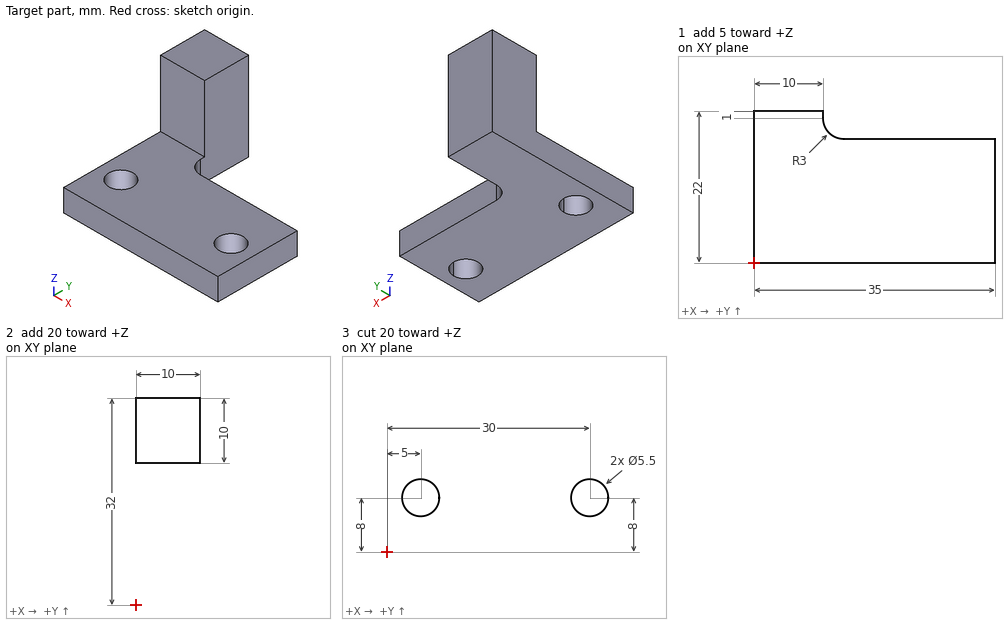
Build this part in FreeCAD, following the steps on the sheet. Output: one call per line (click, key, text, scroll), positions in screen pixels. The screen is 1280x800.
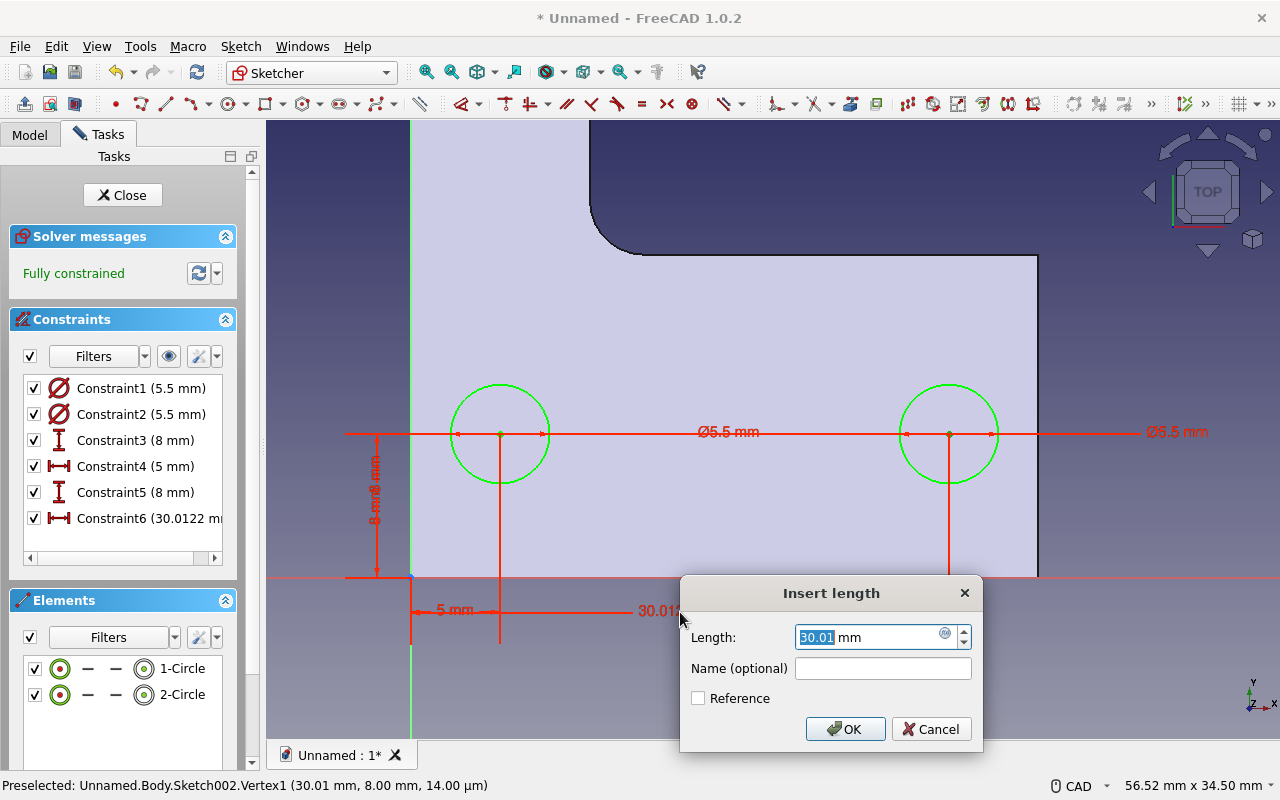
text(30)
key(Return)
key(Escape)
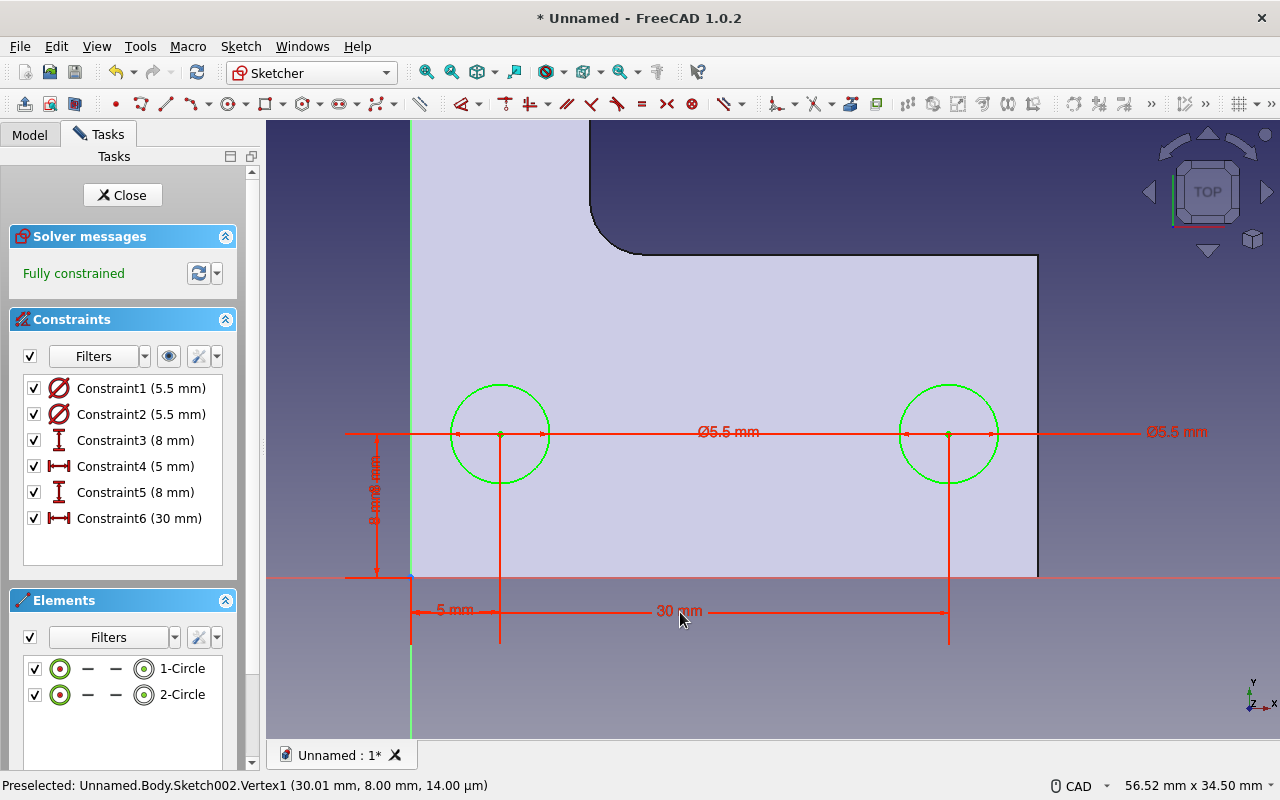
click(123, 195)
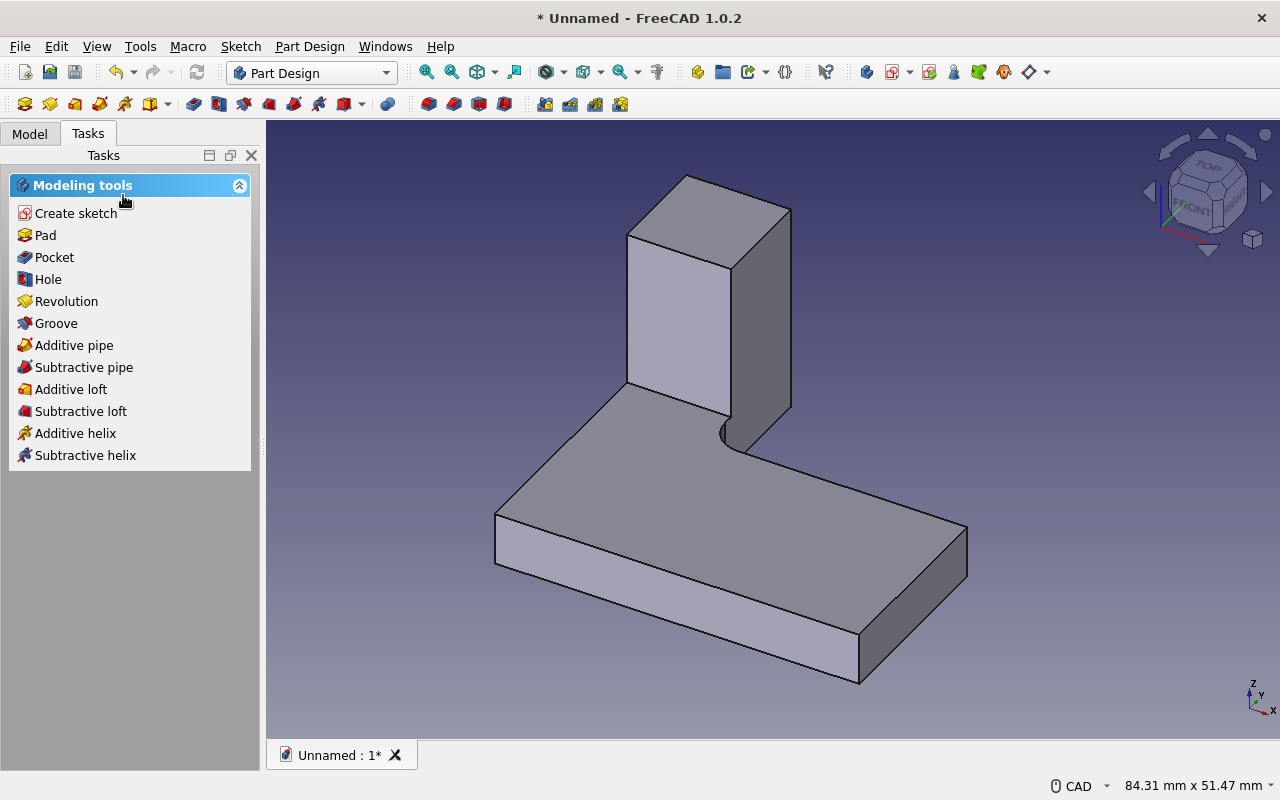
click(194, 104)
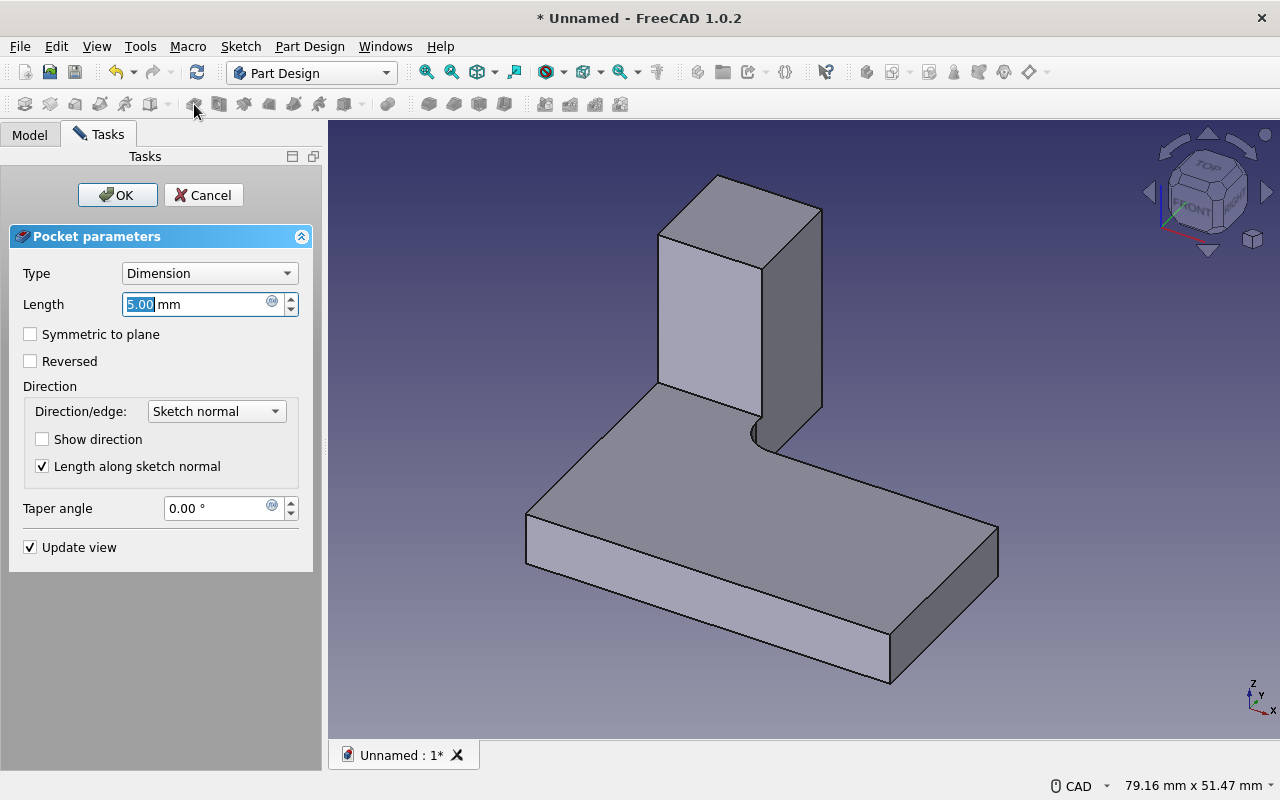
text(20)
key(Tab)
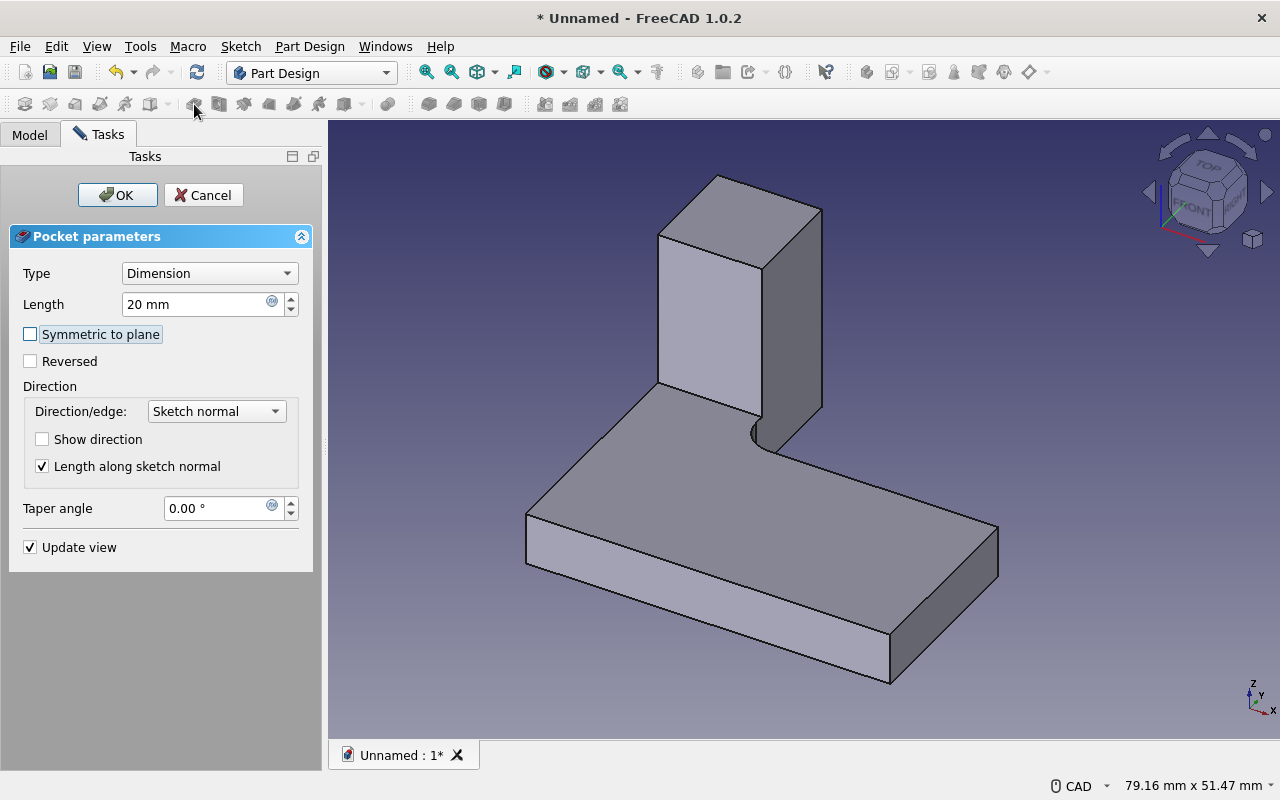
click(31, 361)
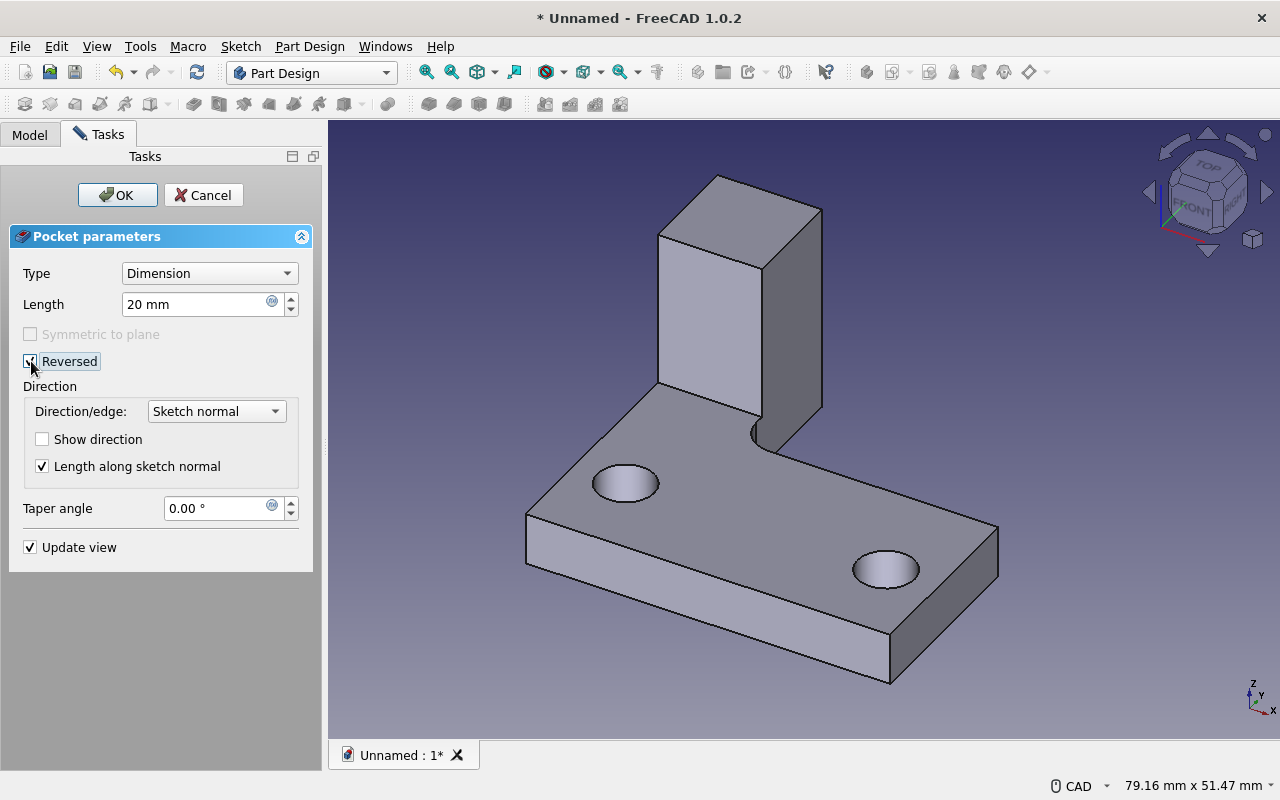
click(118, 195)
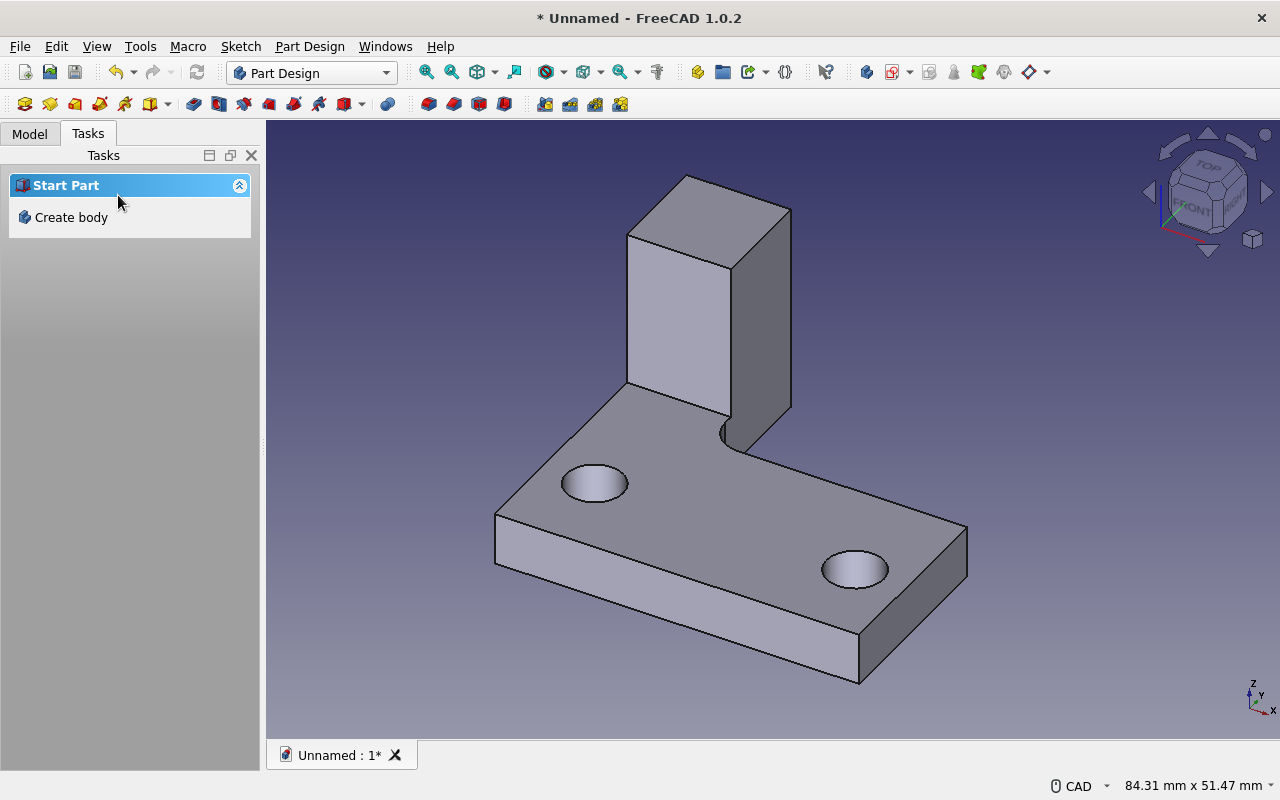
key(0)